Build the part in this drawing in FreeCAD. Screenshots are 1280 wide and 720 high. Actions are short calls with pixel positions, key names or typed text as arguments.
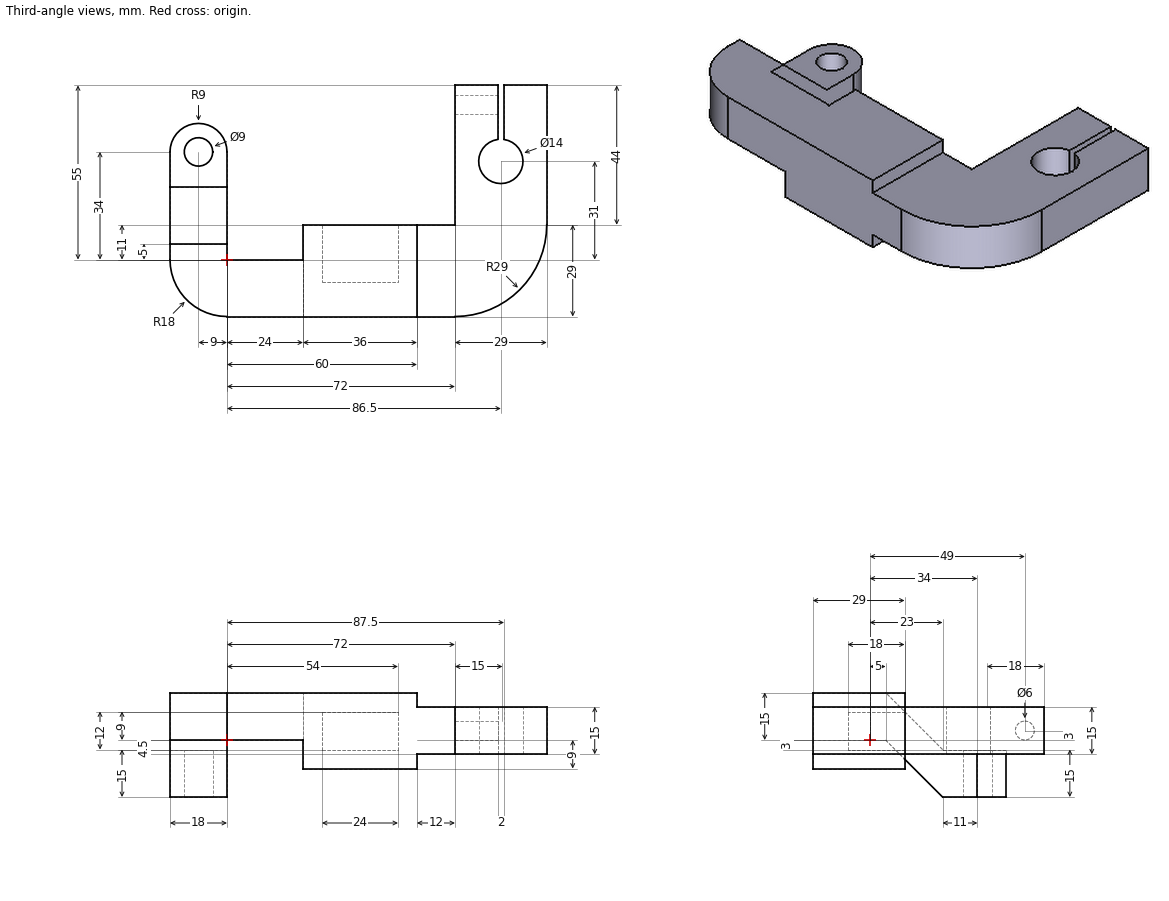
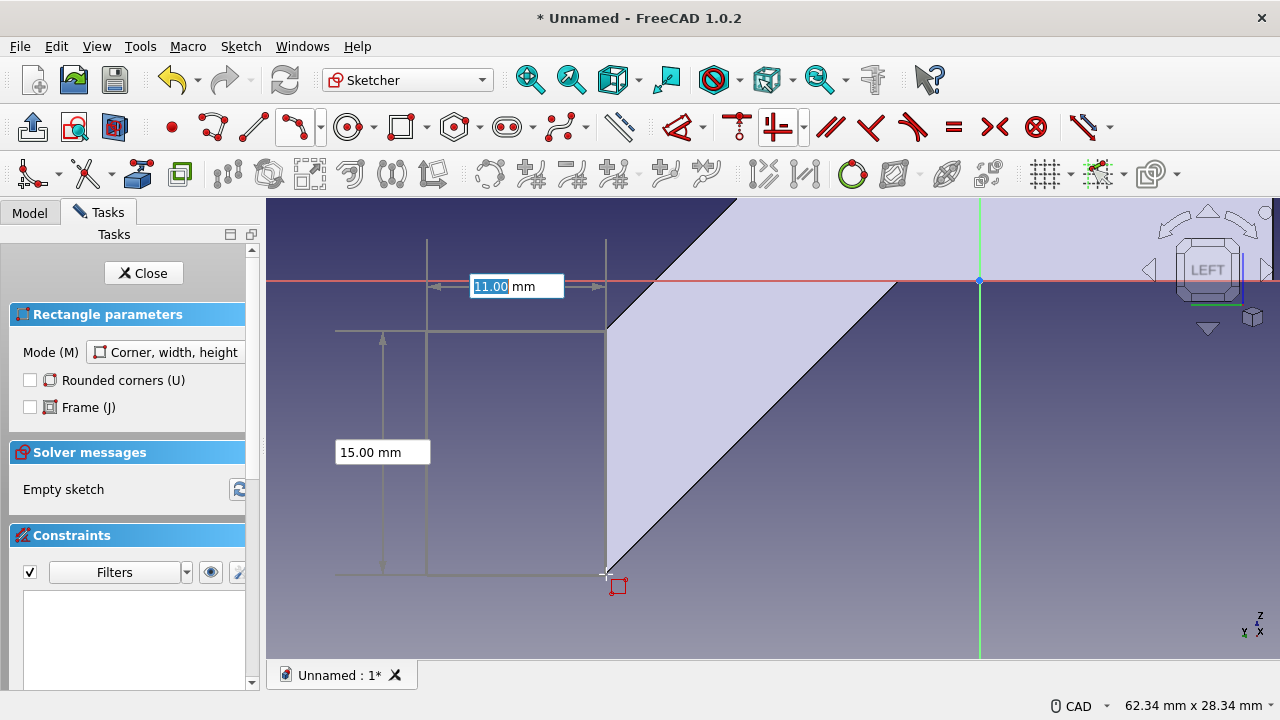
text(11)
key(Tab)
text(15)
key(Return)
key(Escape)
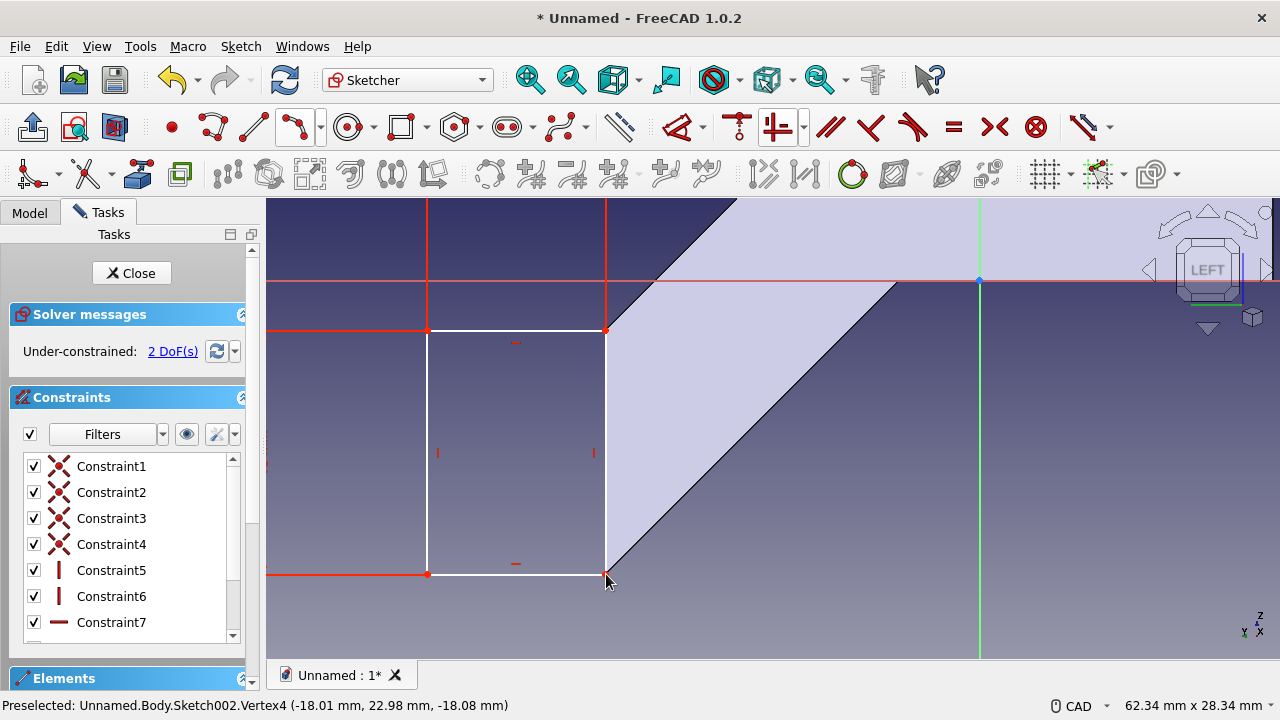
click(676, 128)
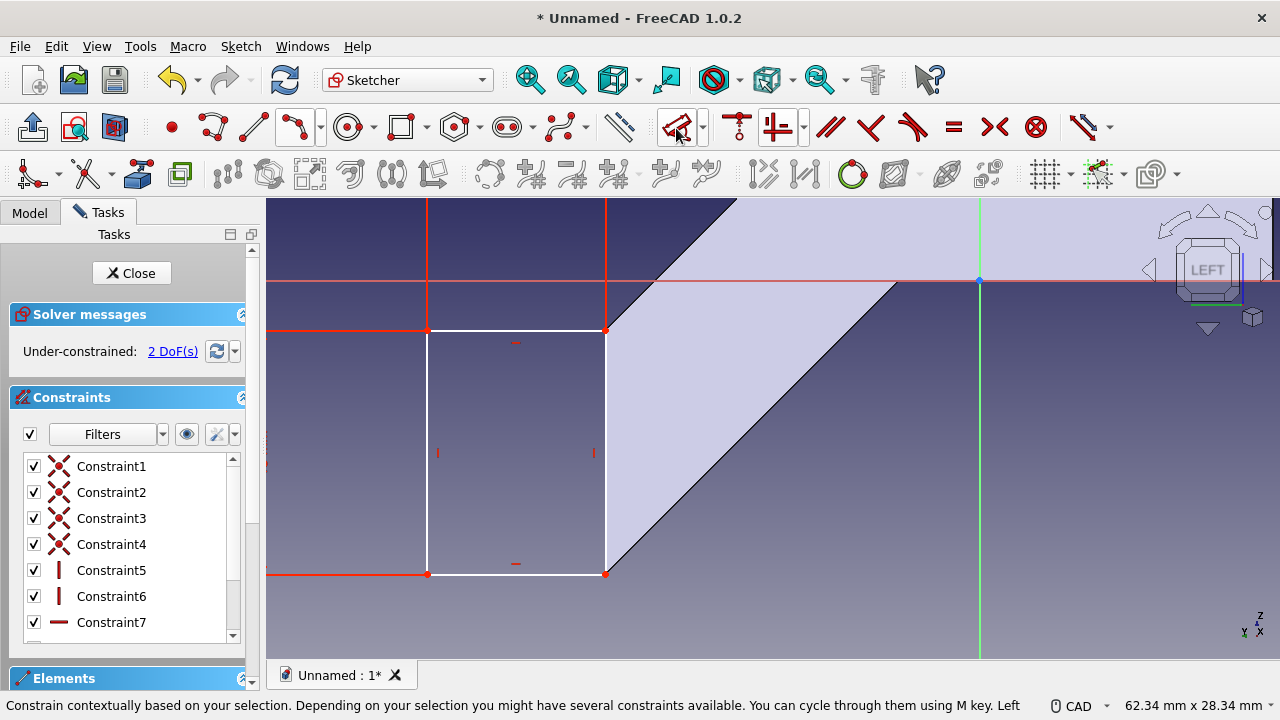
click(427, 331)
click(1014, 306)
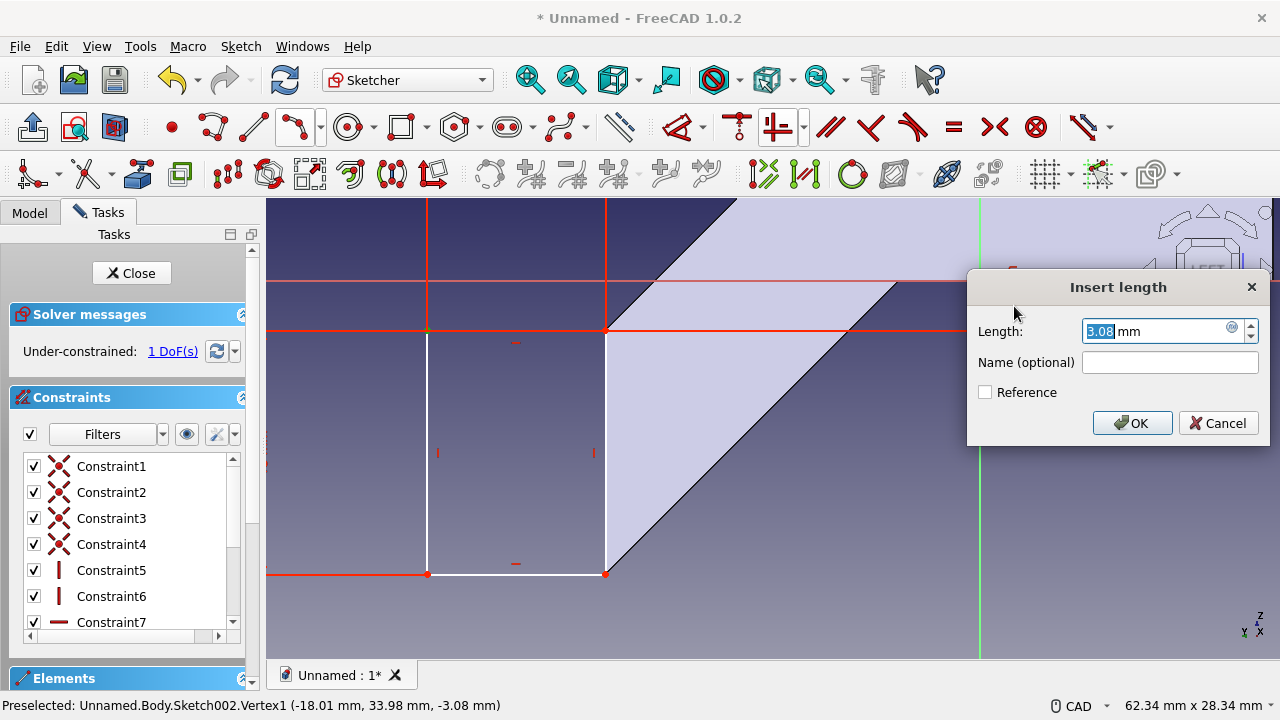
text(3)
key(Return)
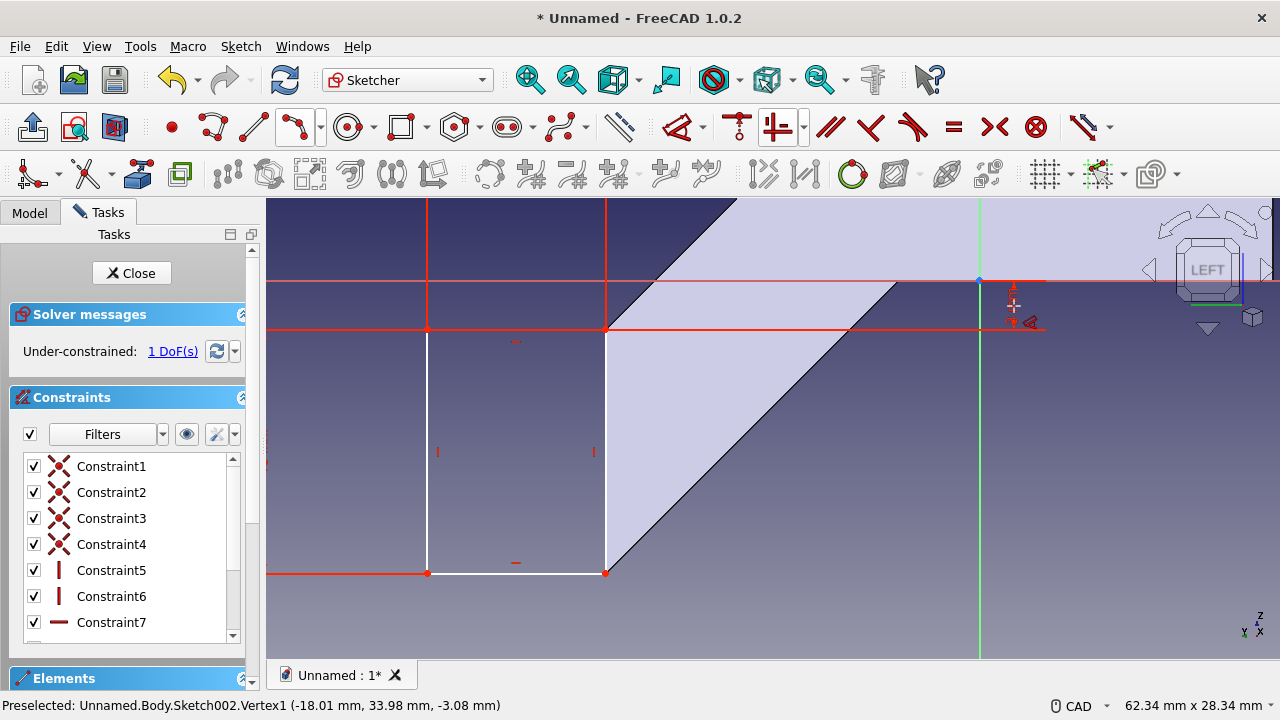
click(427, 330)
click(703, 247)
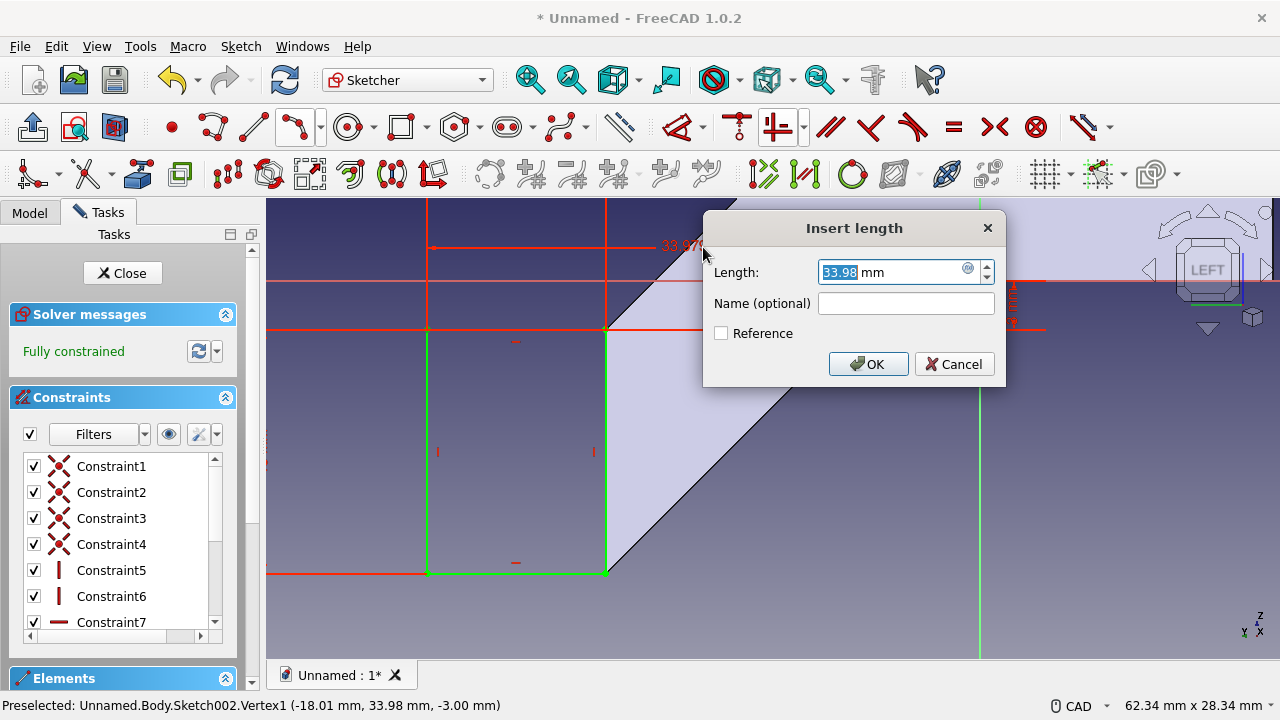
text(34)
key(Return)
key(Escape)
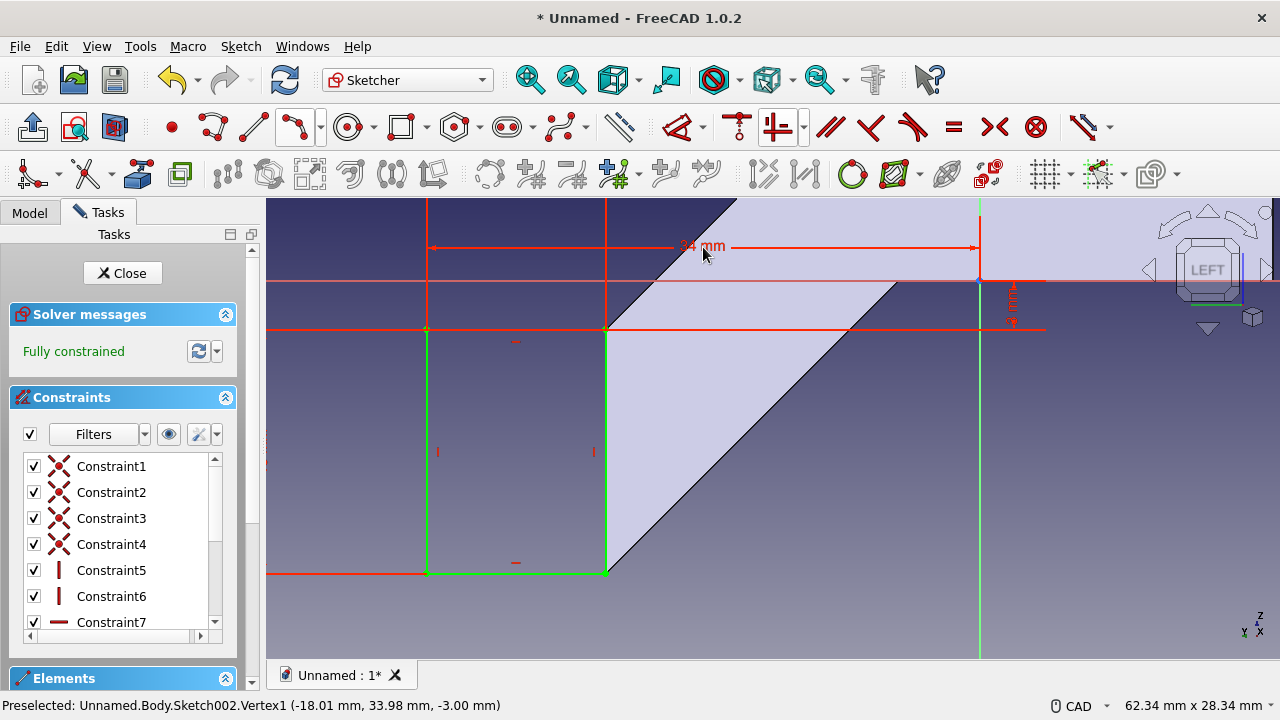
click(123, 273)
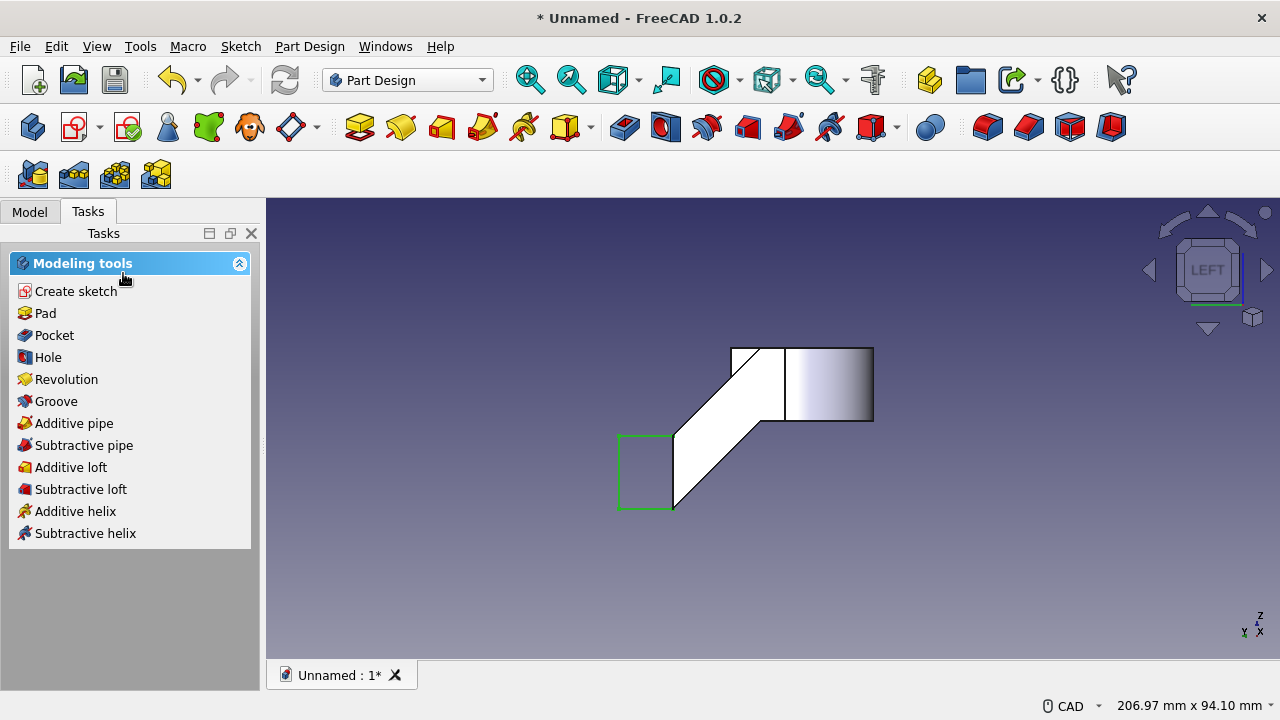
click(360, 128)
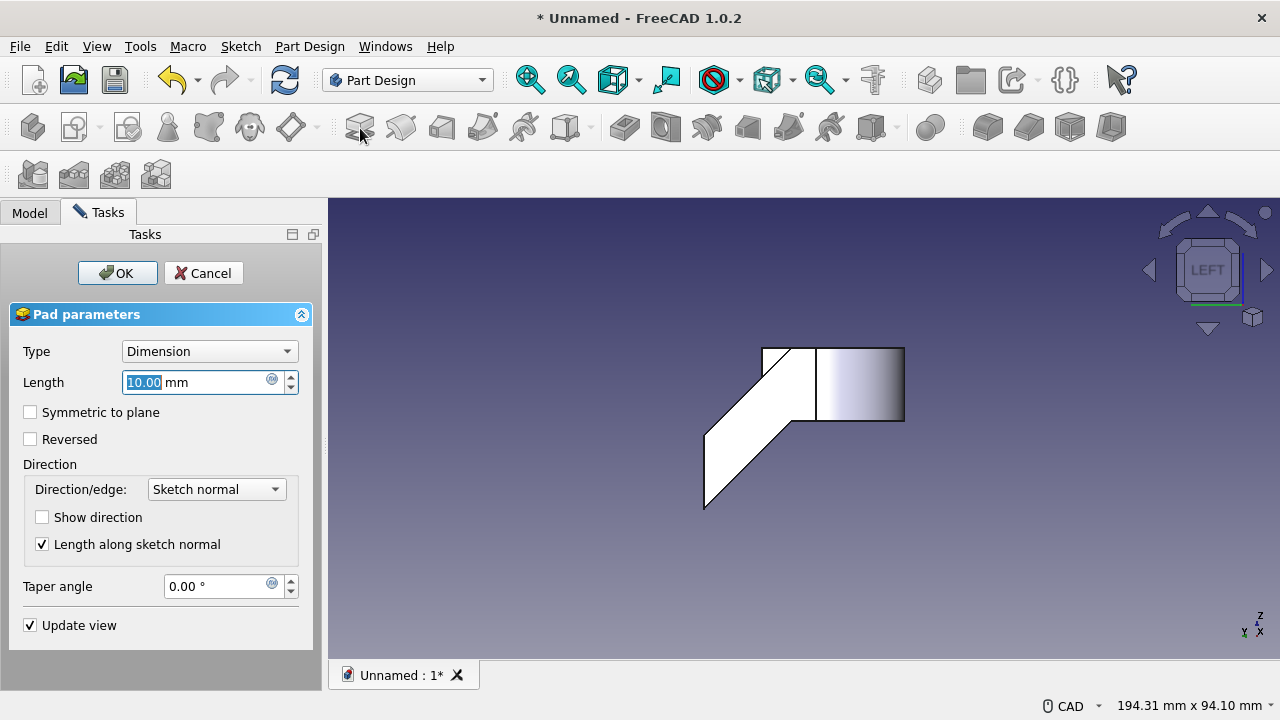
text(18)
key(Tab)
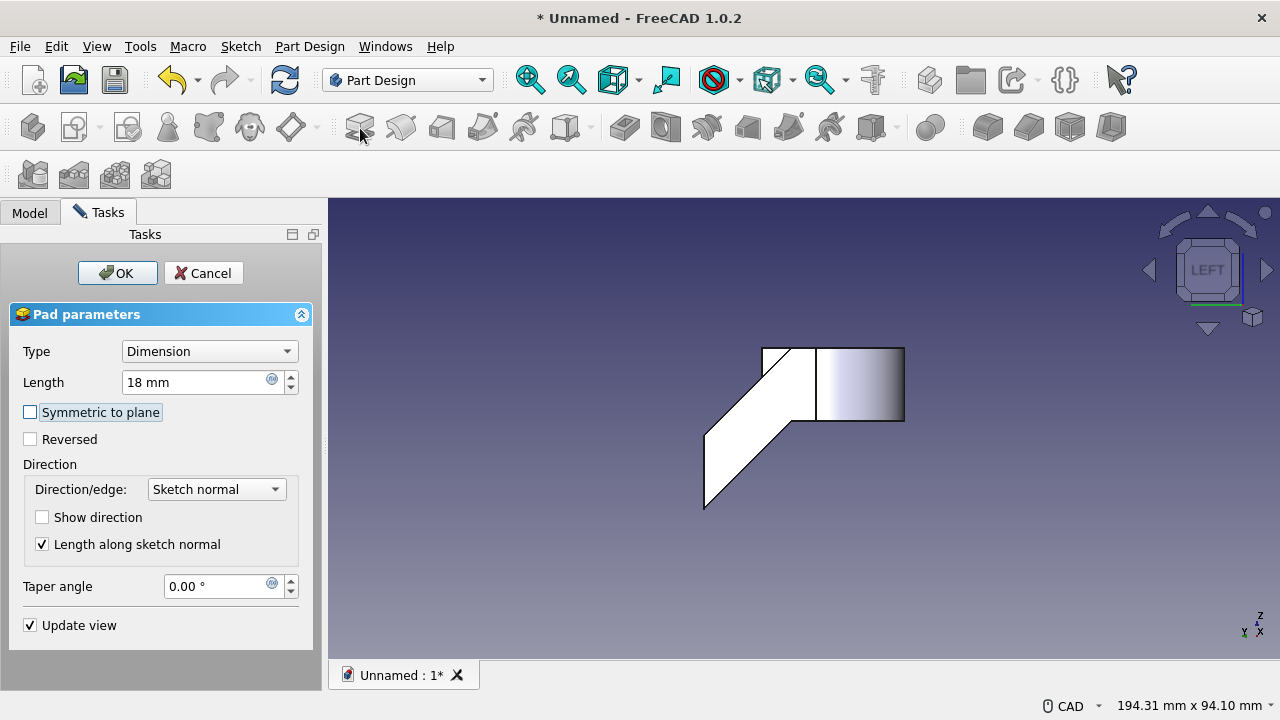
click(31, 439)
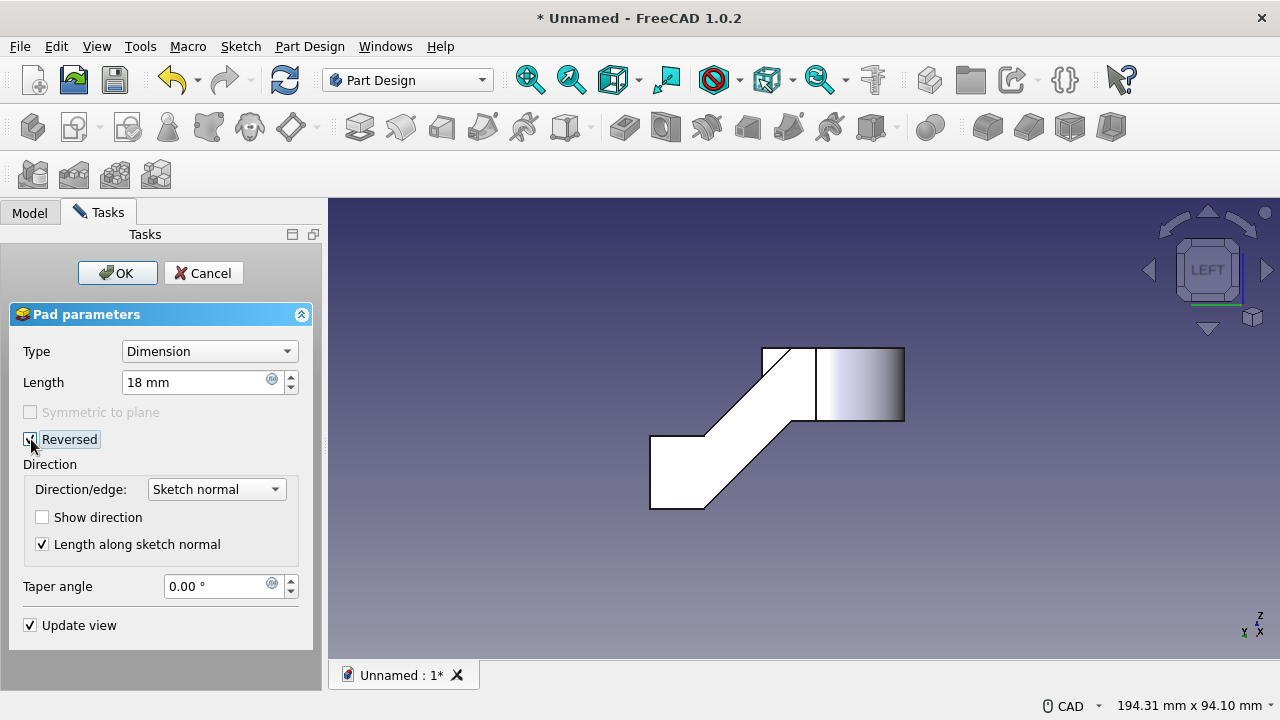
click(118, 273)